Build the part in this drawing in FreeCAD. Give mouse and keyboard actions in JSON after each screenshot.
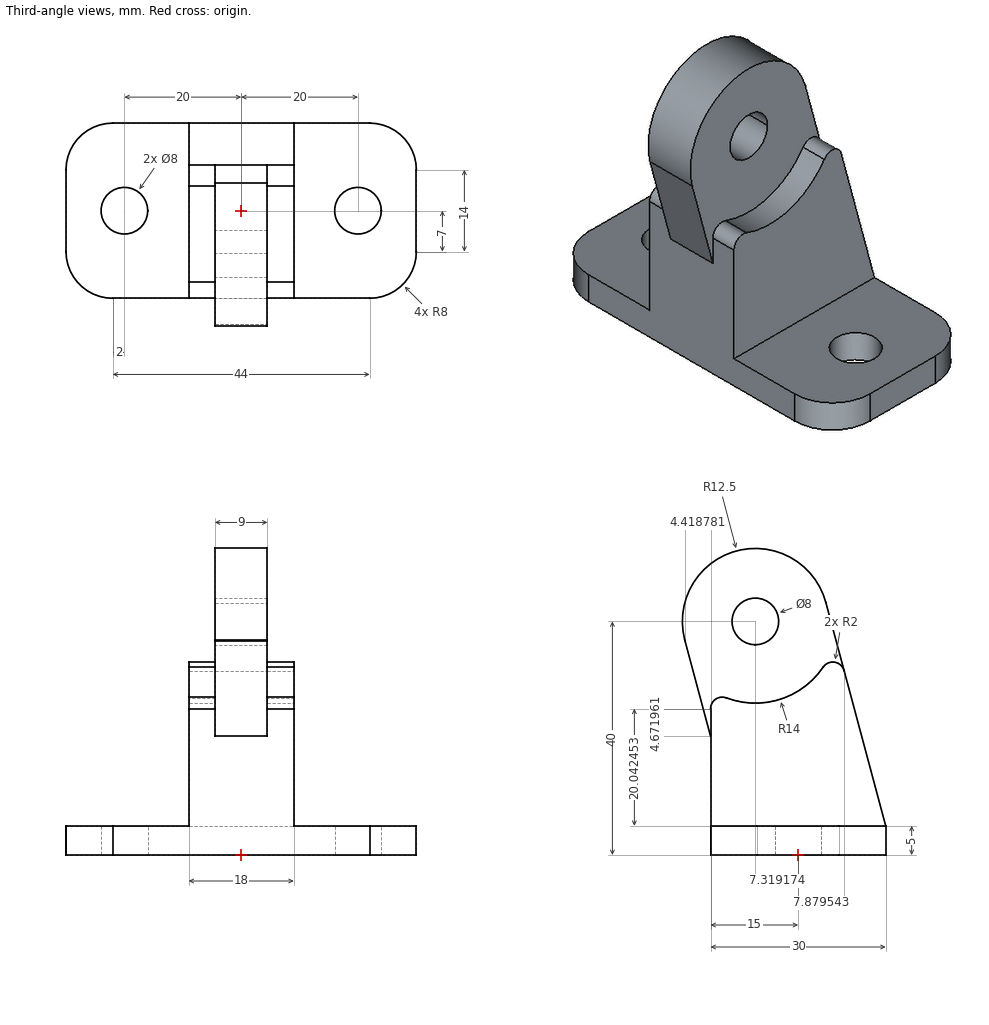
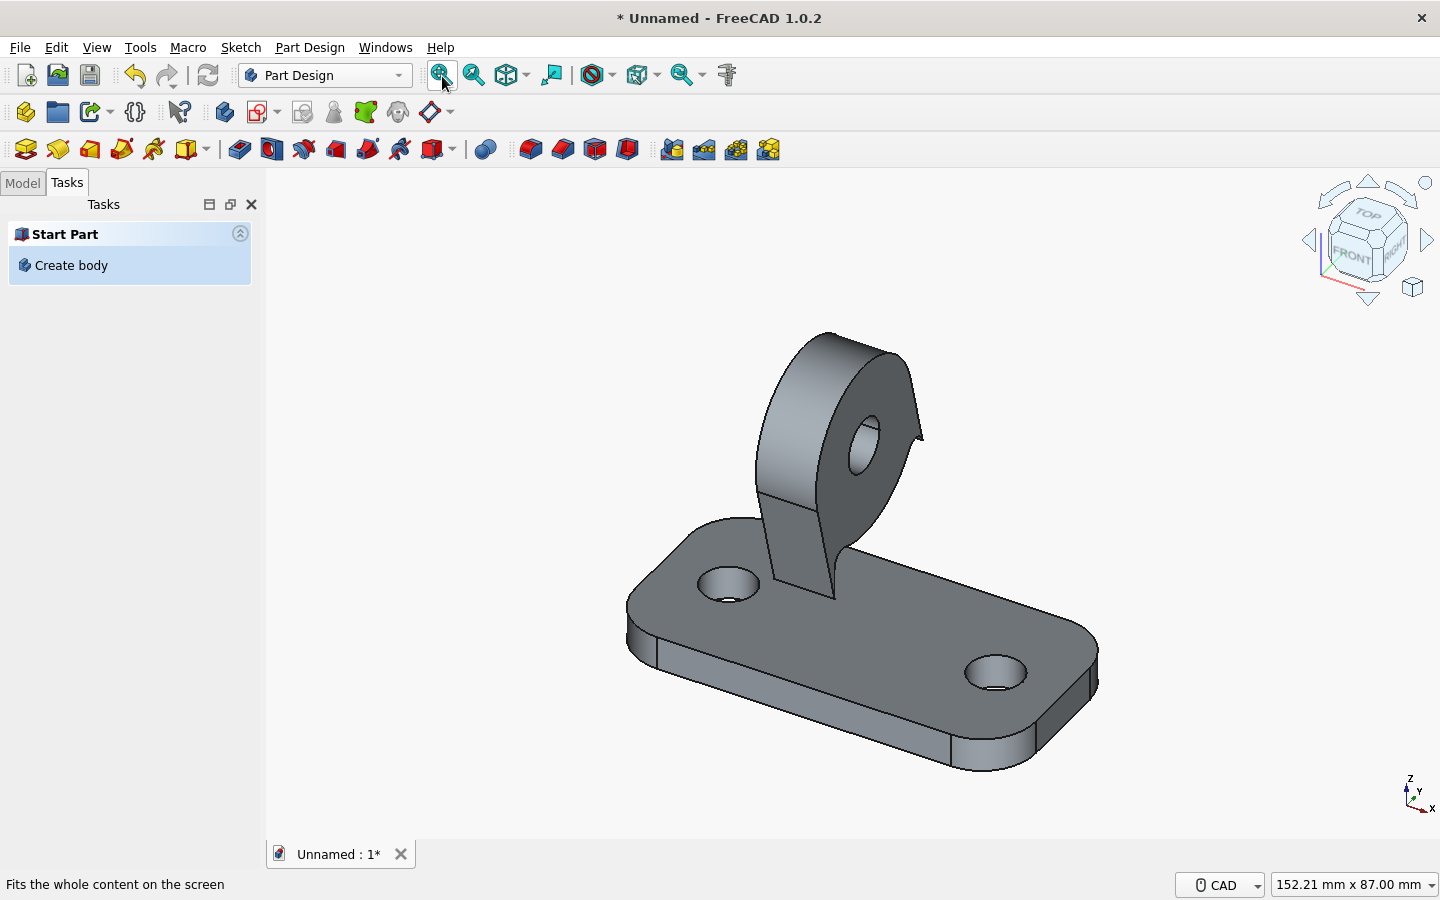
{"action": "left_click", "coordinate": [23, 182]}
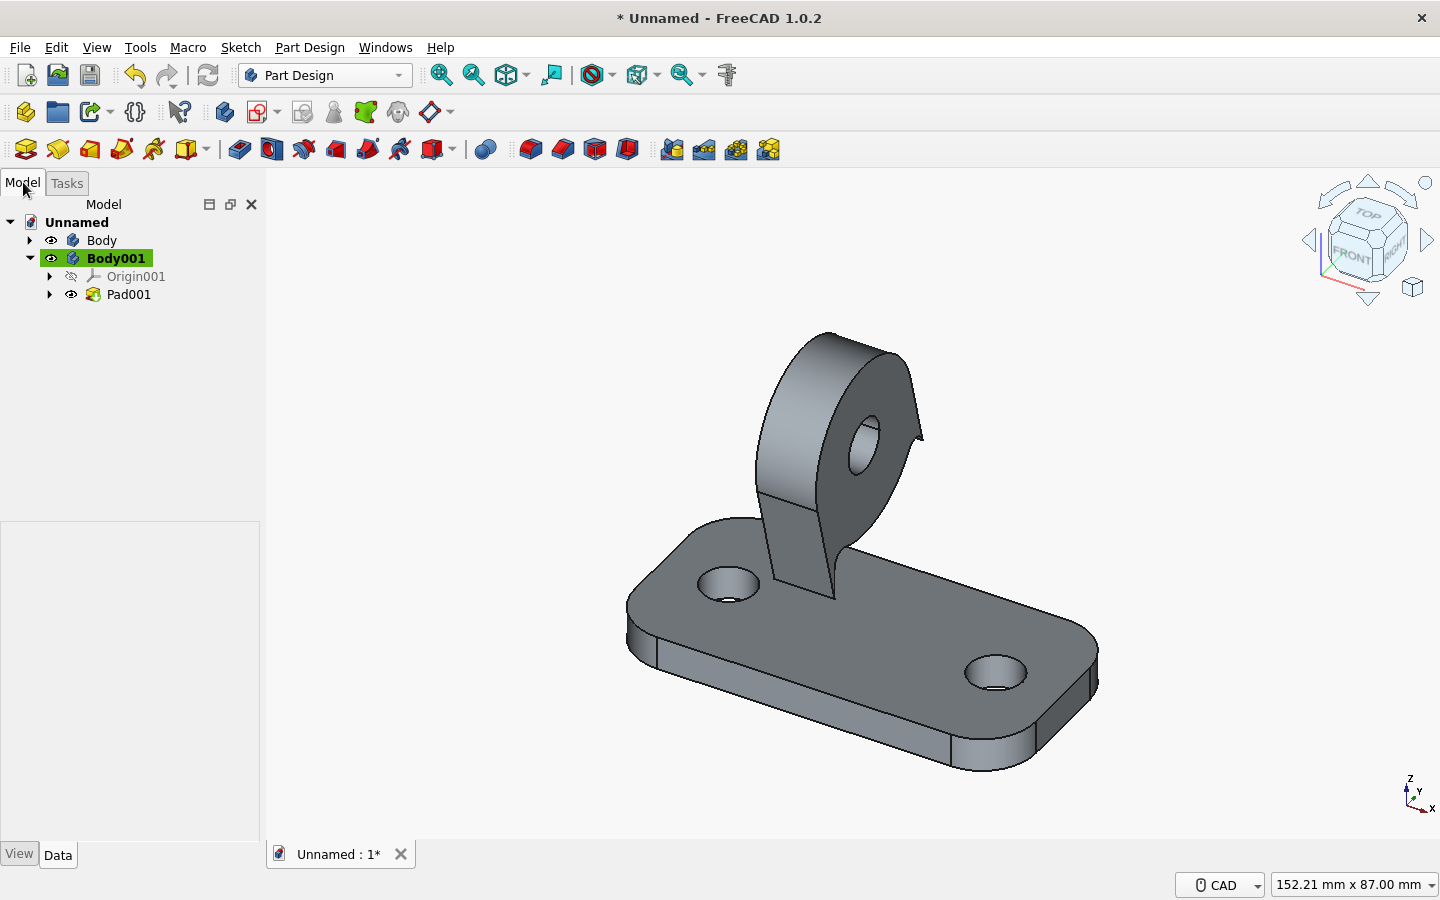
{"action": "double_click", "coordinate": [96, 240]}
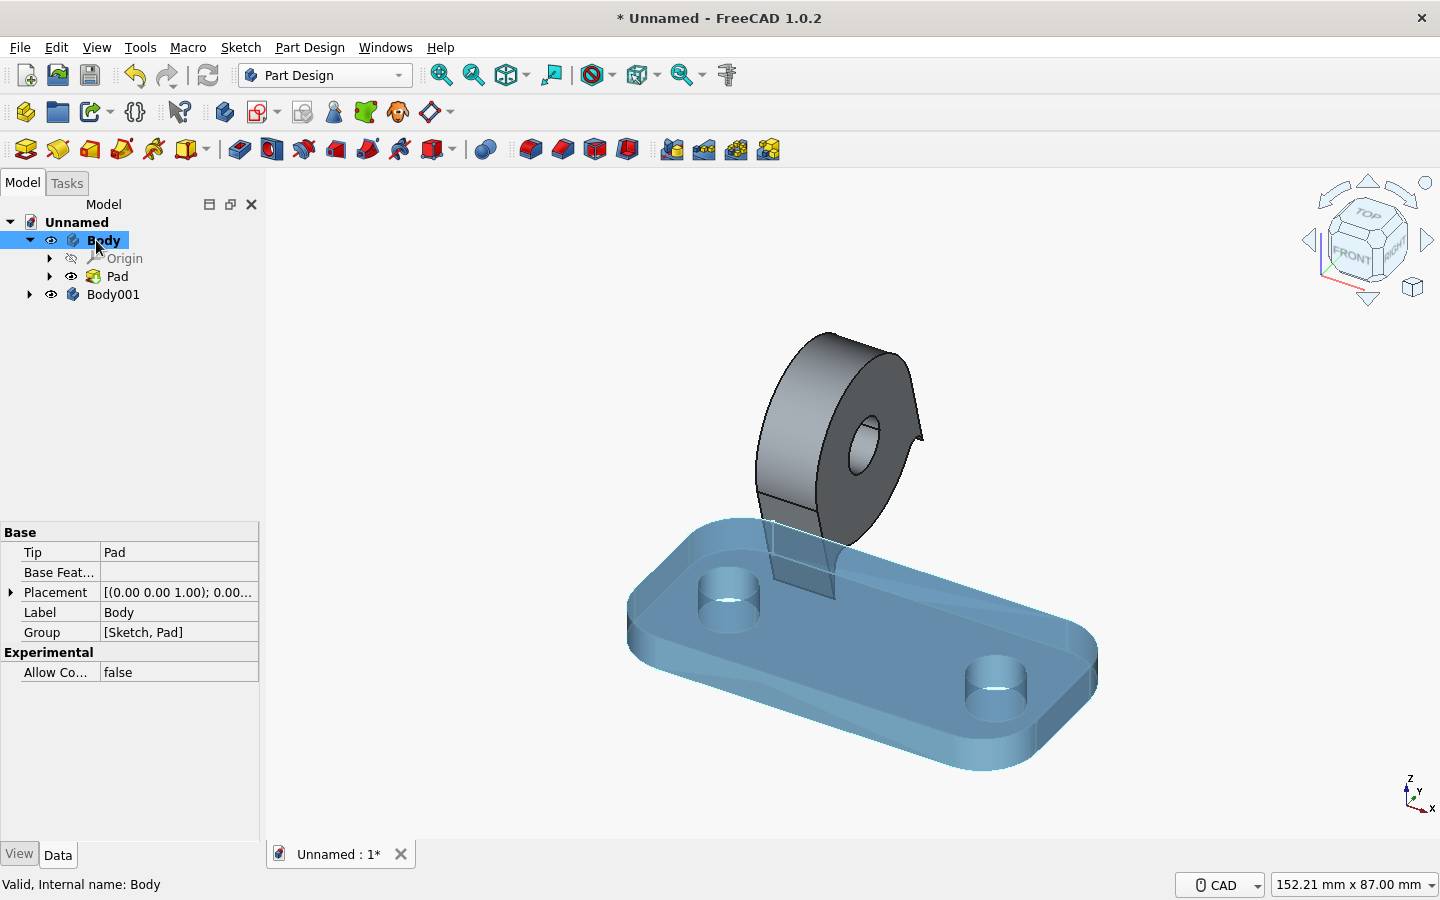
{"action": "left_click", "coordinate": [96, 240]}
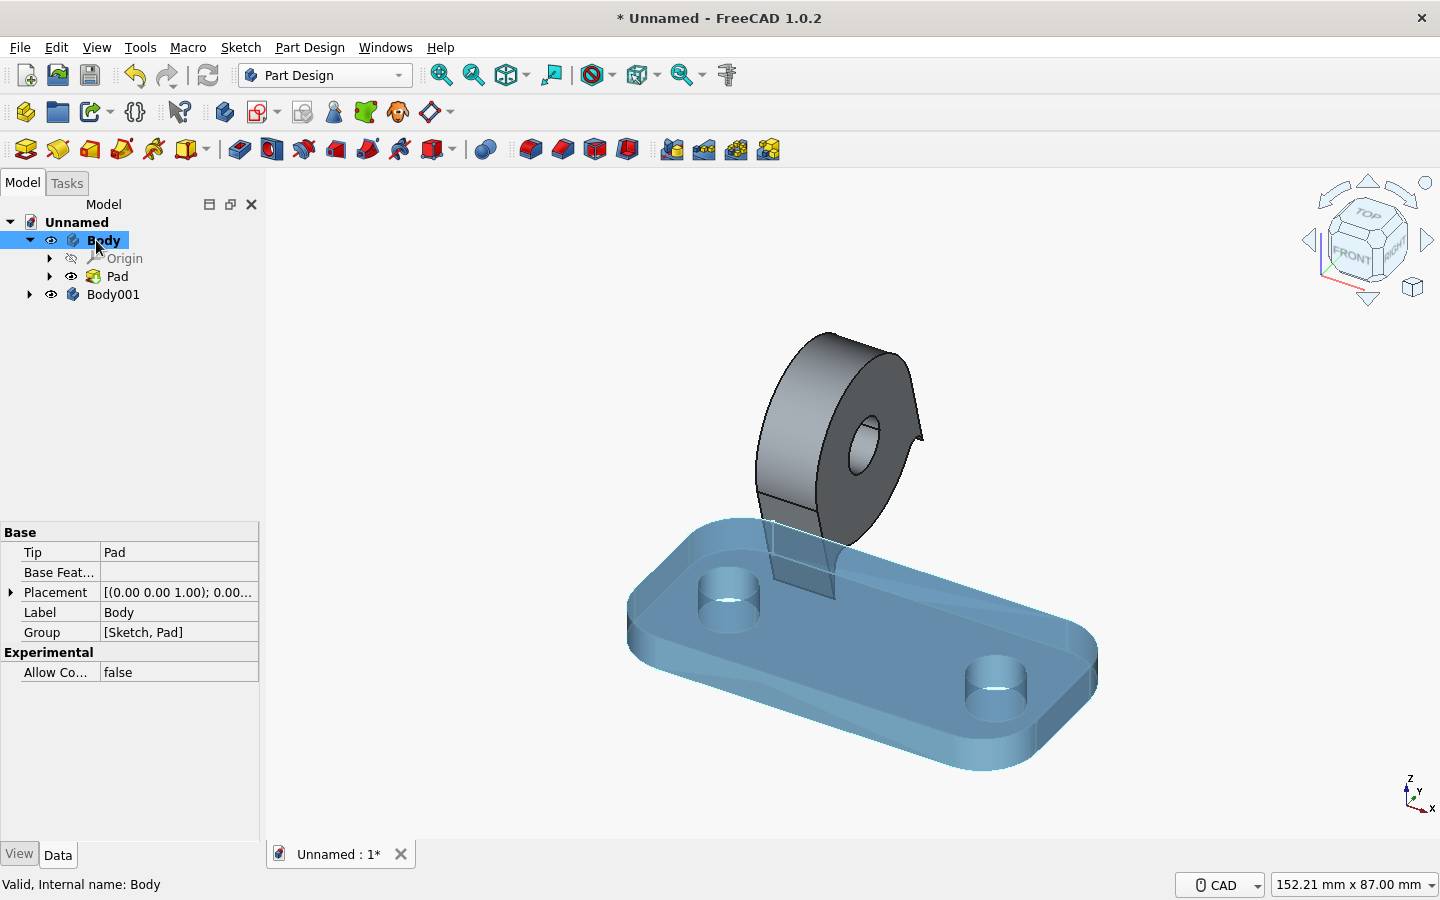
{"action": "left_click", "coordinate": [146, 672]}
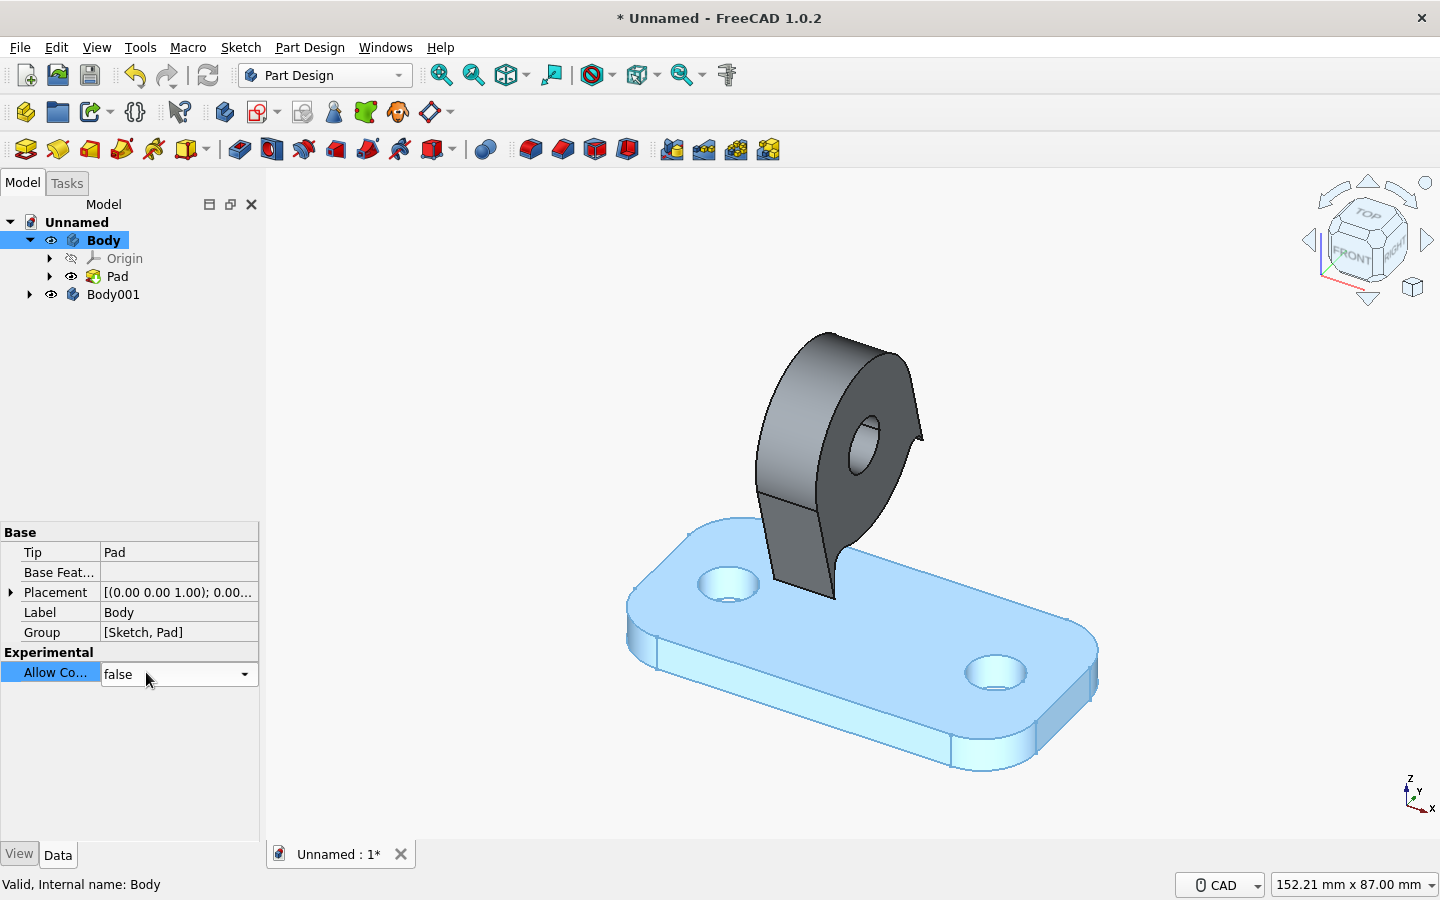
{"action": "left_click", "coordinate": [146, 672]}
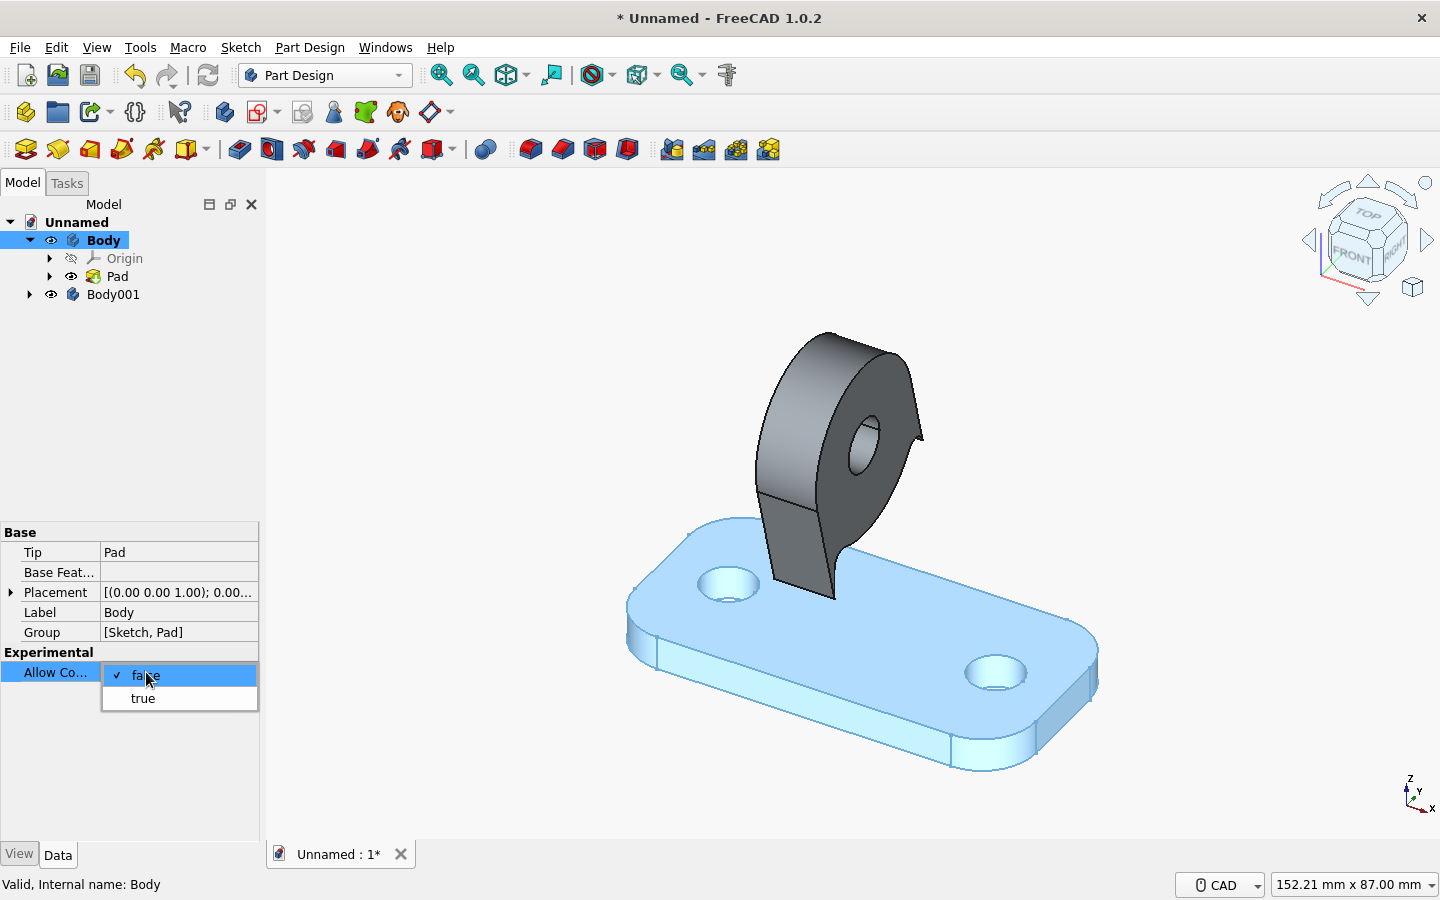
{"action": "left_click", "coordinate": [179, 698]}
{"action": "key", "text": "Return"}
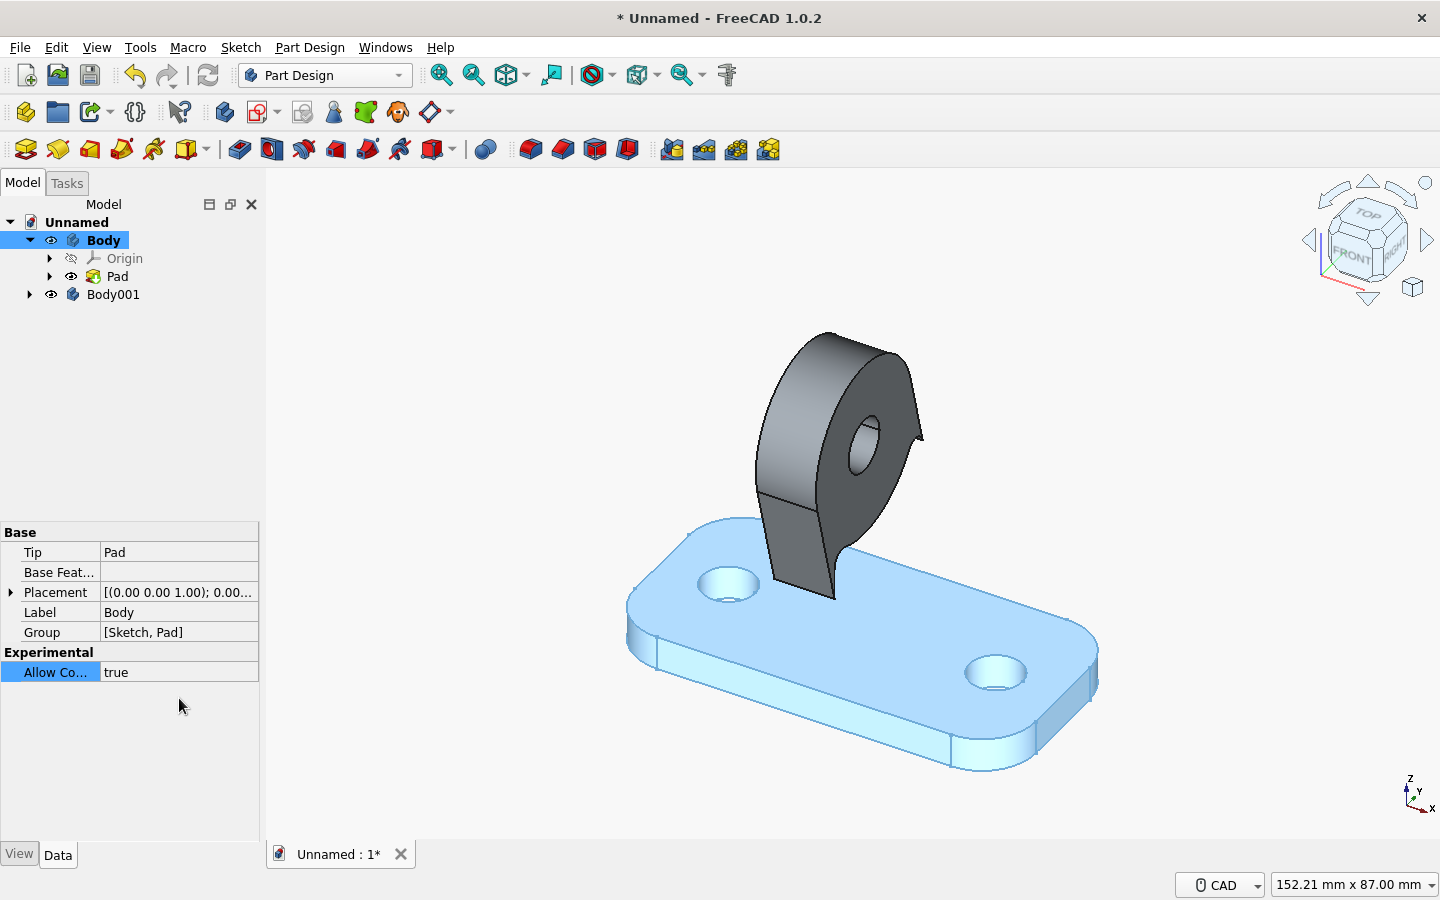
{"action": "left_click", "coordinate": [96, 294]}